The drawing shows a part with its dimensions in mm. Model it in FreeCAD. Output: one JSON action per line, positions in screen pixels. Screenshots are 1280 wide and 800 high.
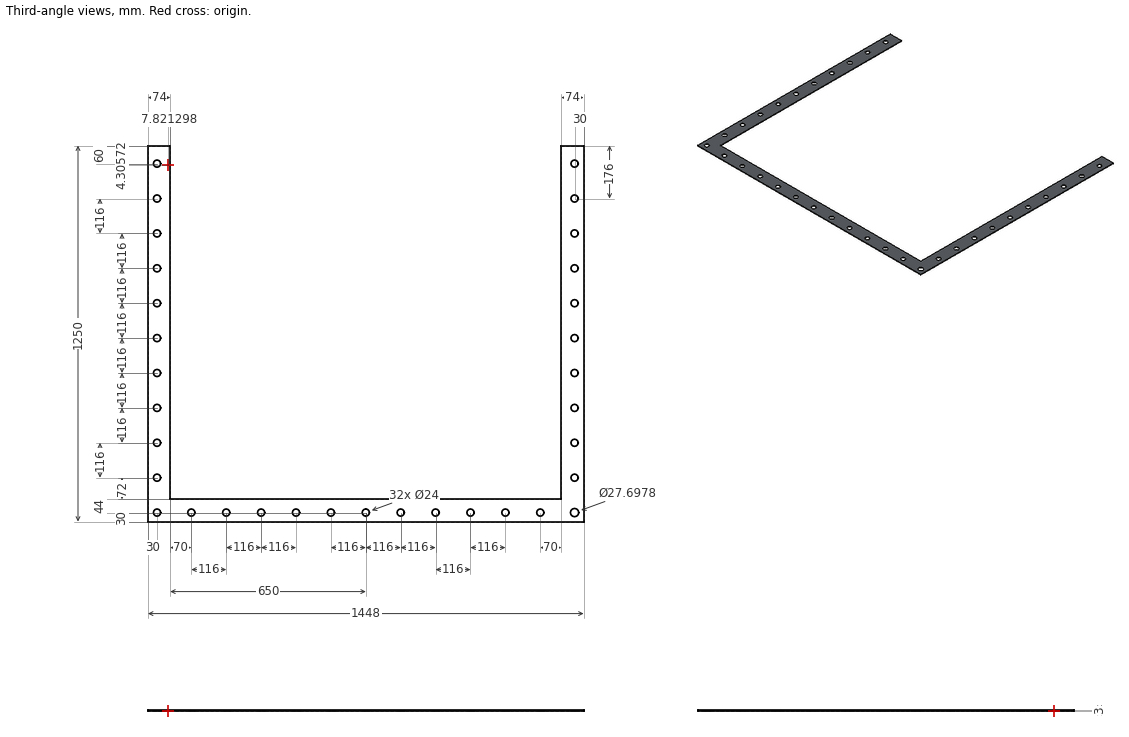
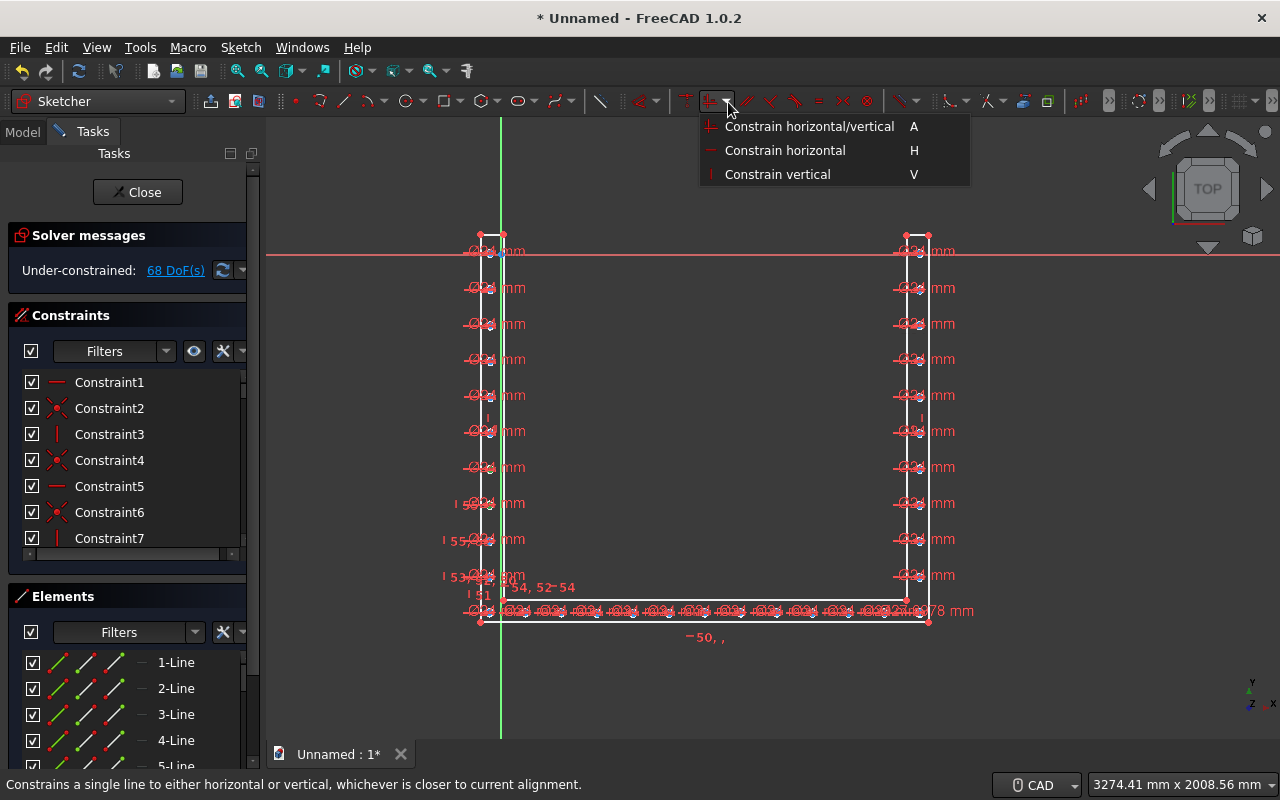
{"action": "left_click", "coordinate": [835, 174]}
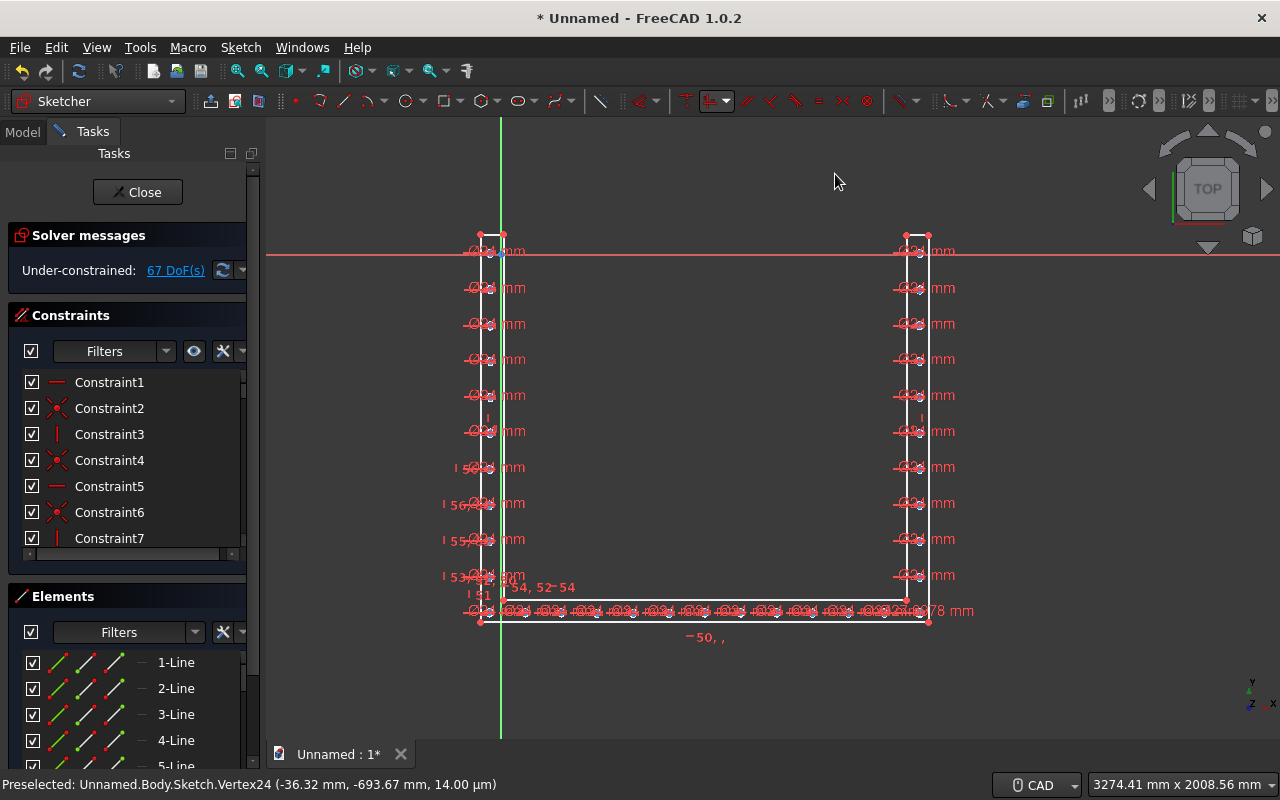
{"action": "left_click", "coordinate": [561, 613]}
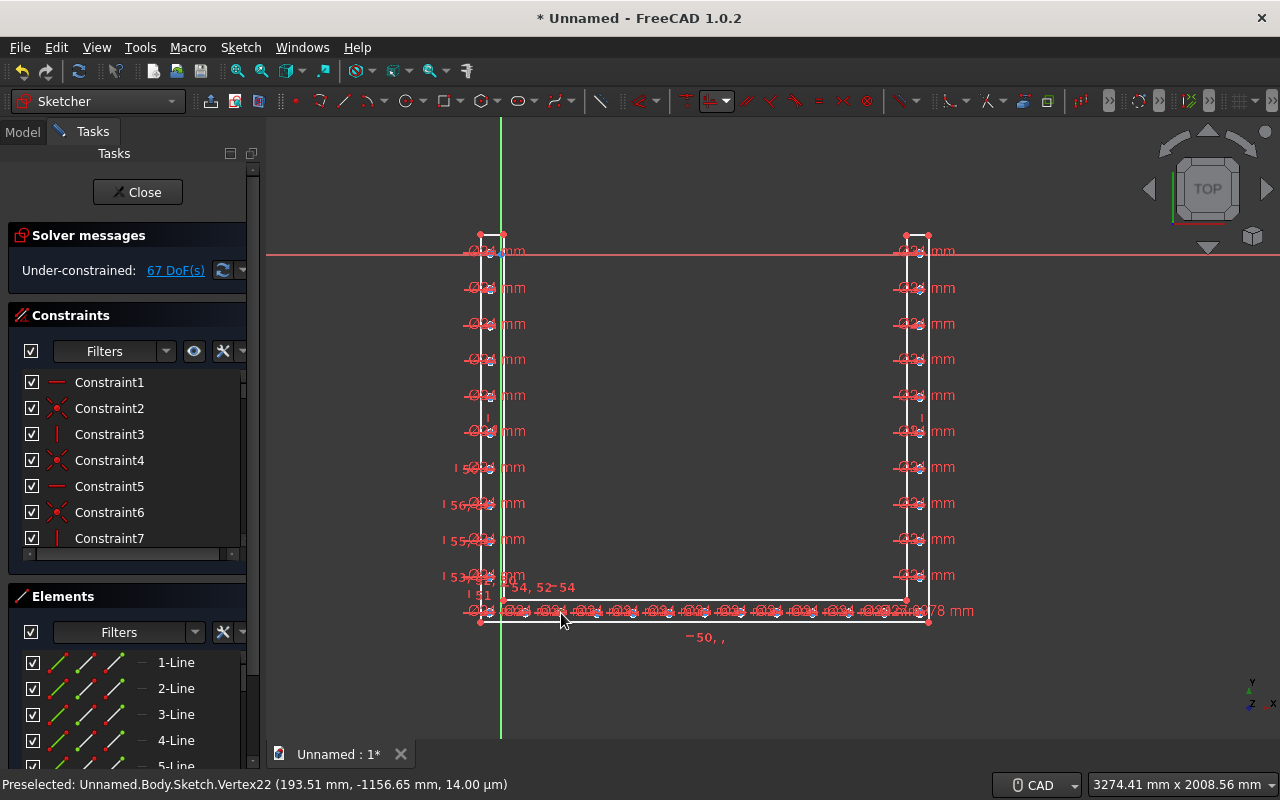
{"action": "left_click", "coordinate": [597, 613]}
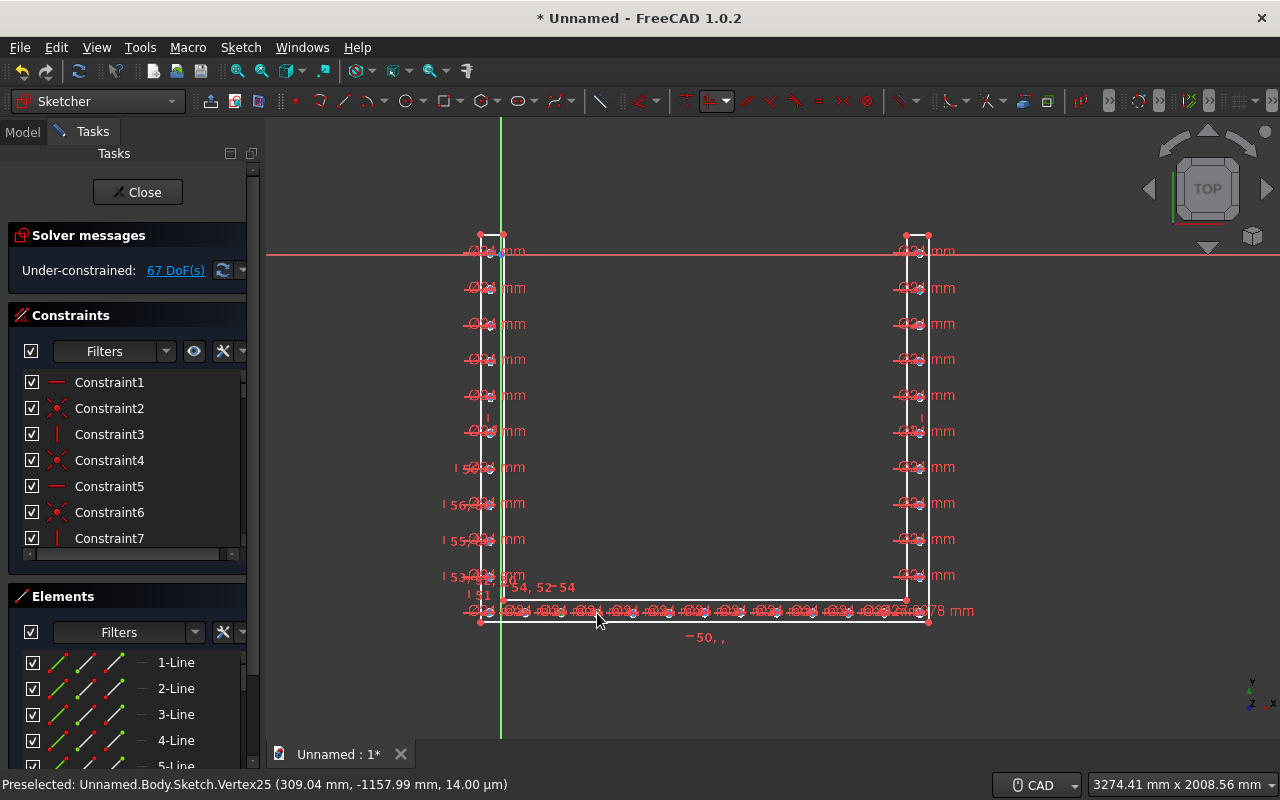
{"action": "left_click", "coordinate": [728, 102]}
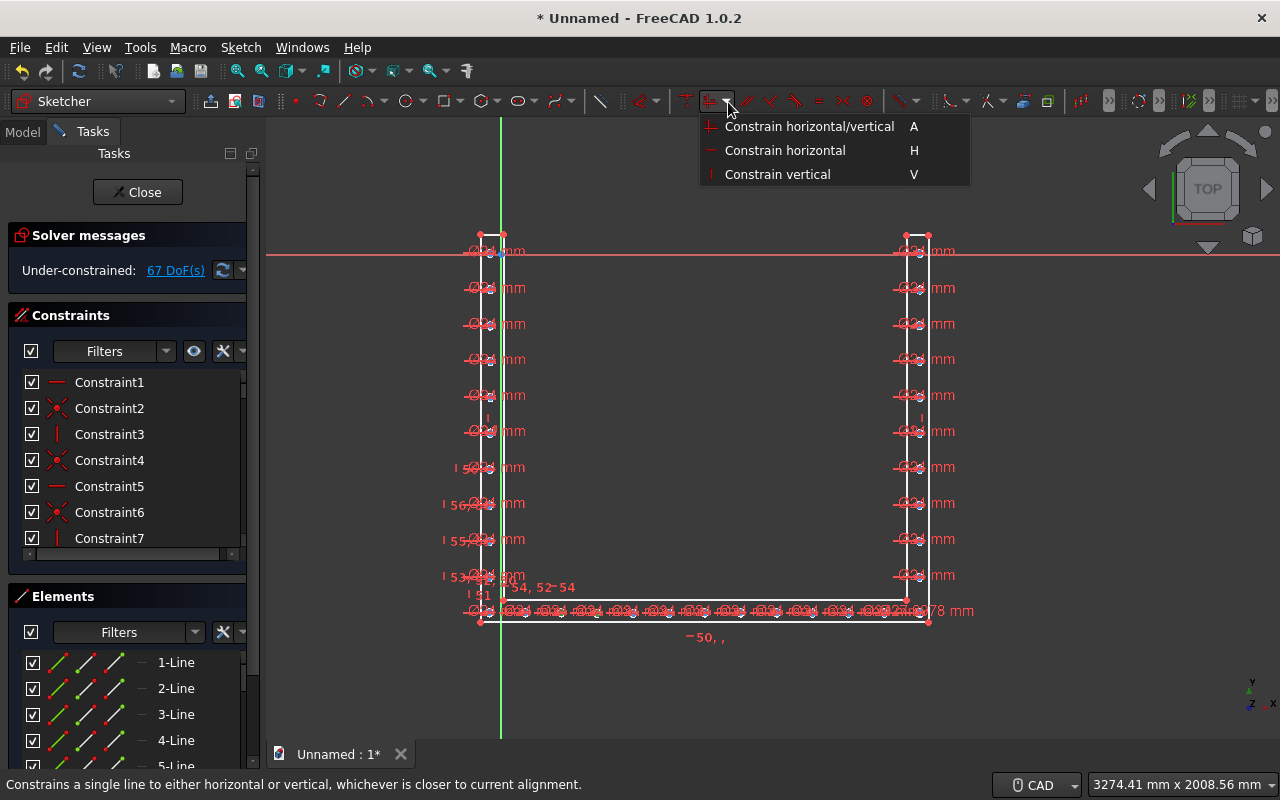
{"action": "left_click", "coordinate": [835, 150]}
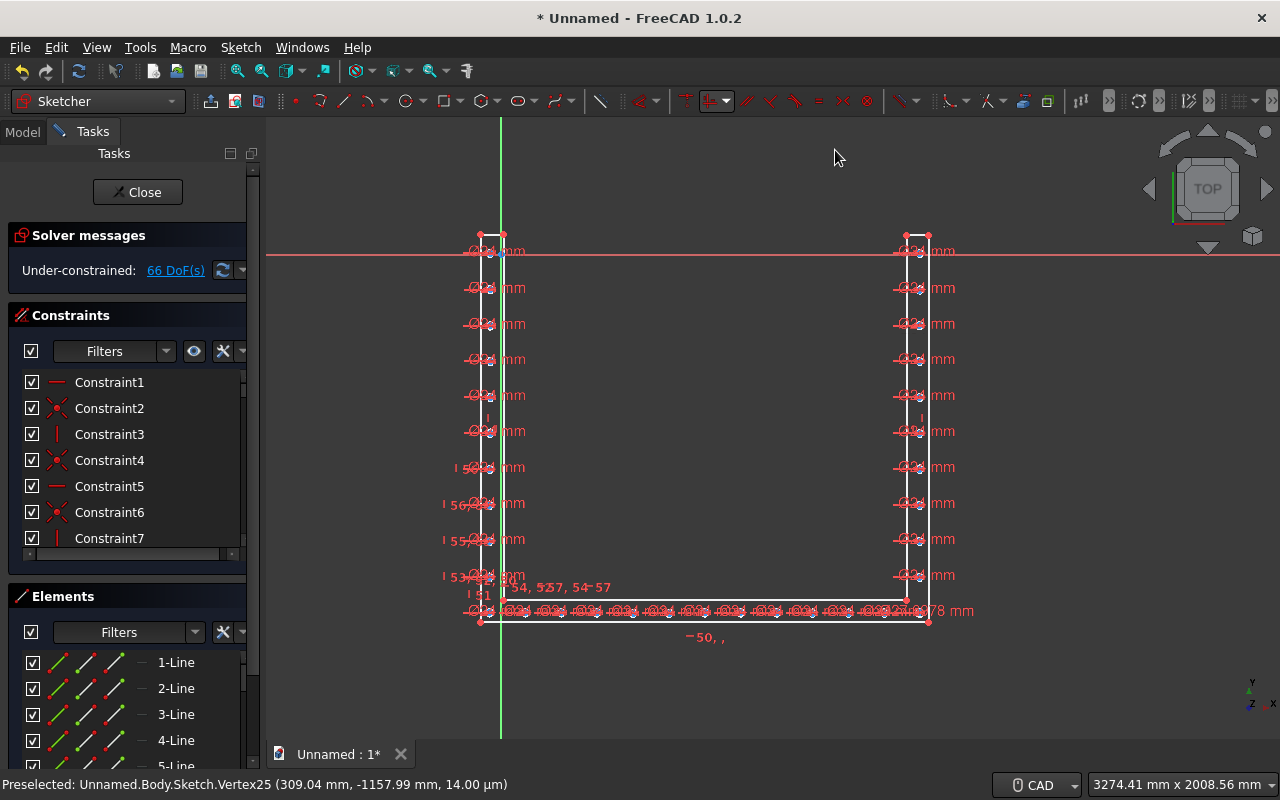
{"action": "left_click", "coordinate": [597, 613]}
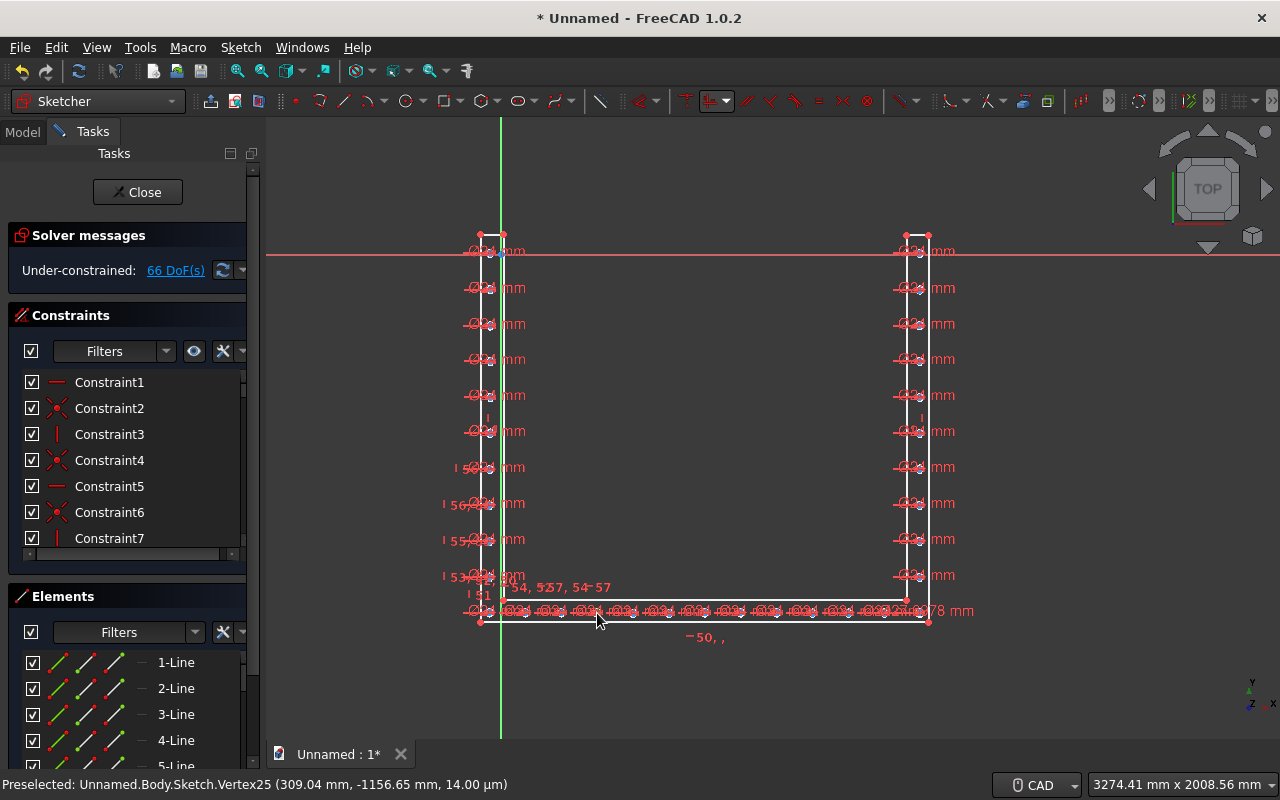
{"action": "left_click", "coordinate": [633, 613]}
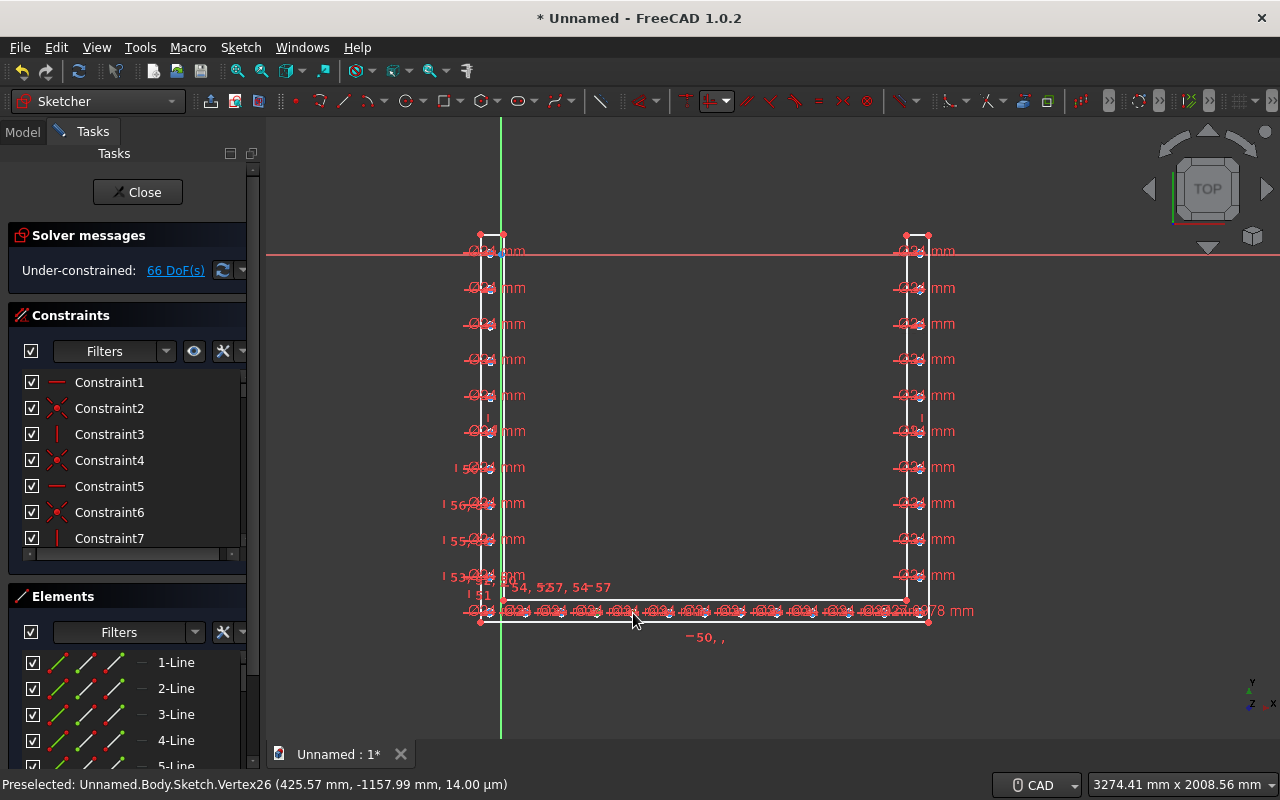
{"action": "left_click", "coordinate": [728, 102]}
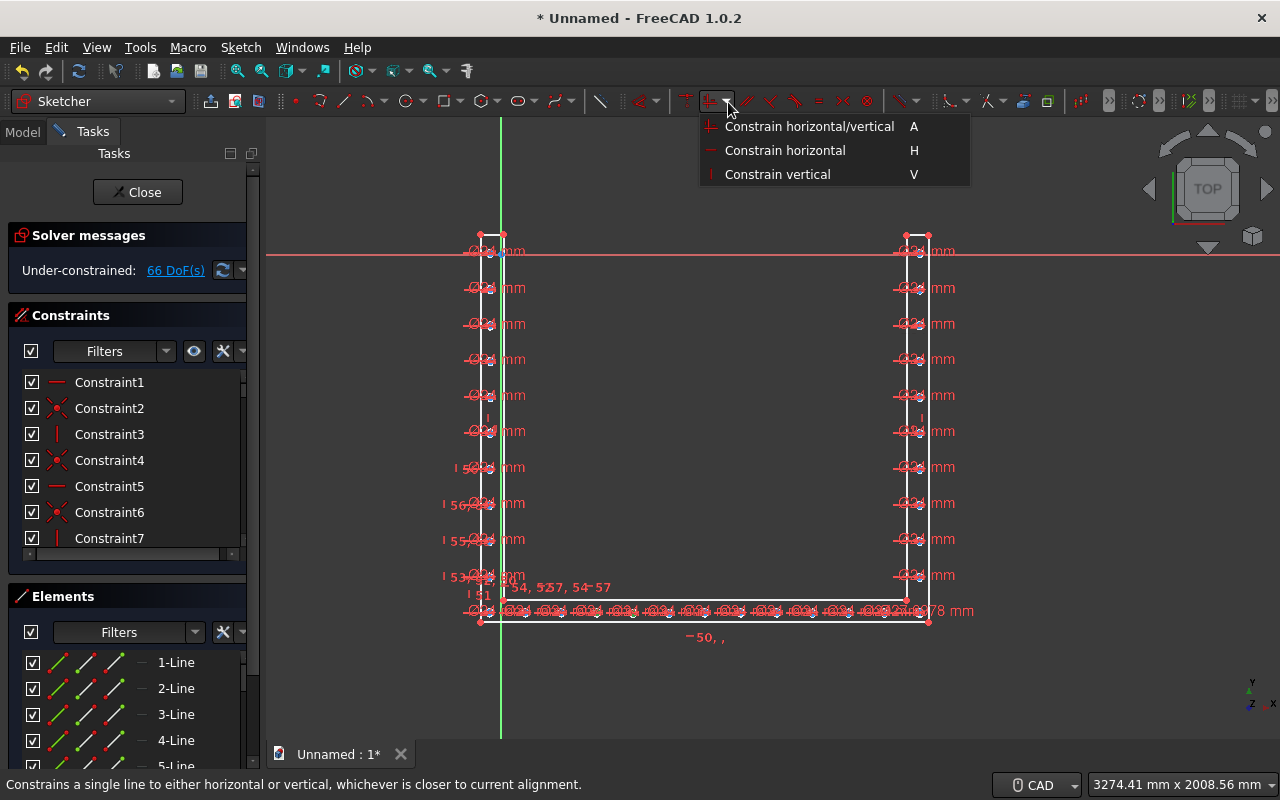
{"action": "left_click", "coordinate": [835, 150]}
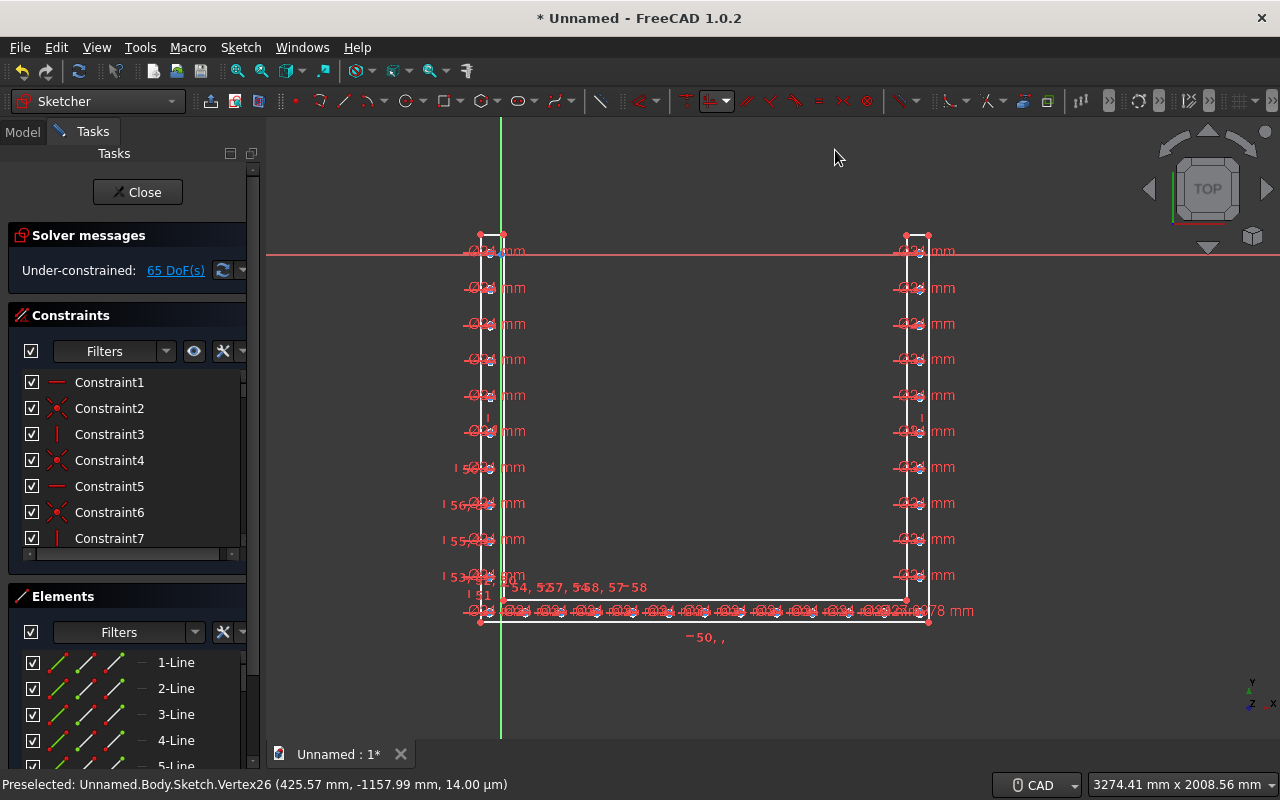
{"action": "left_click", "coordinate": [705, 613]}